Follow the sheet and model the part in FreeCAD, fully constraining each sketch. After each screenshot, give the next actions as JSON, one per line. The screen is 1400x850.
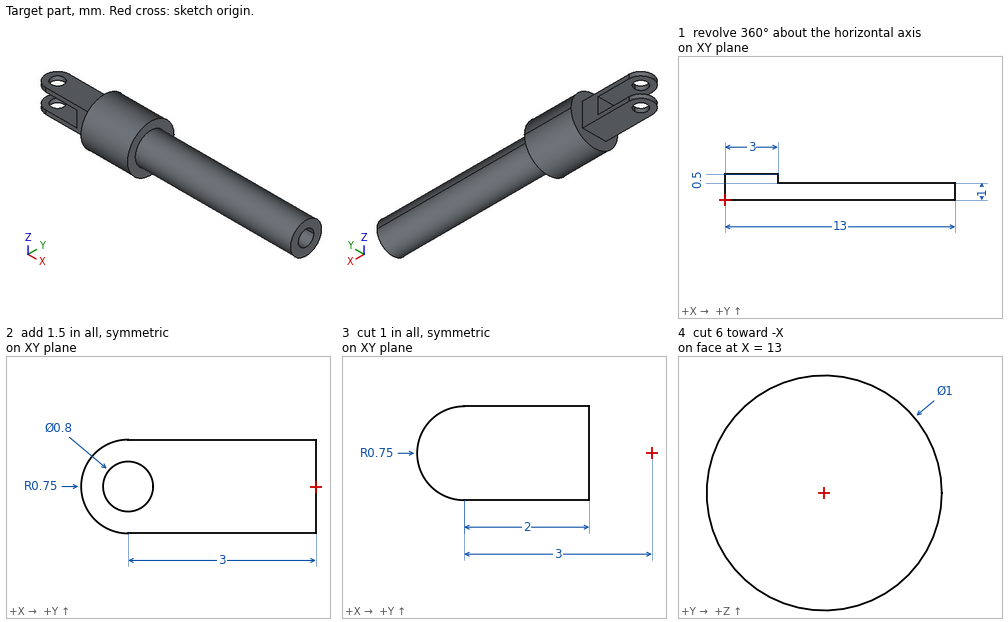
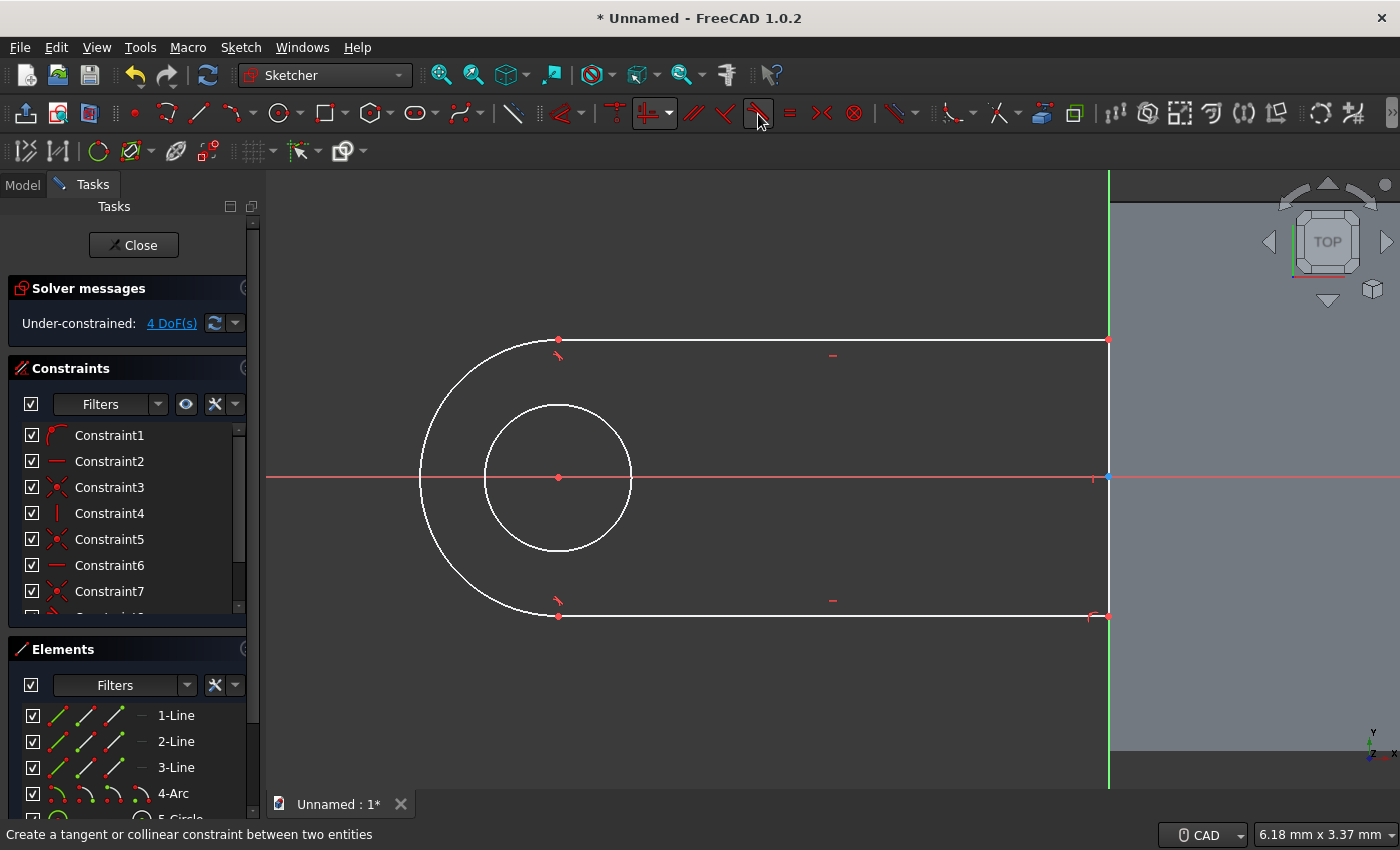
{"action": "left_click", "coordinate": [558, 478]}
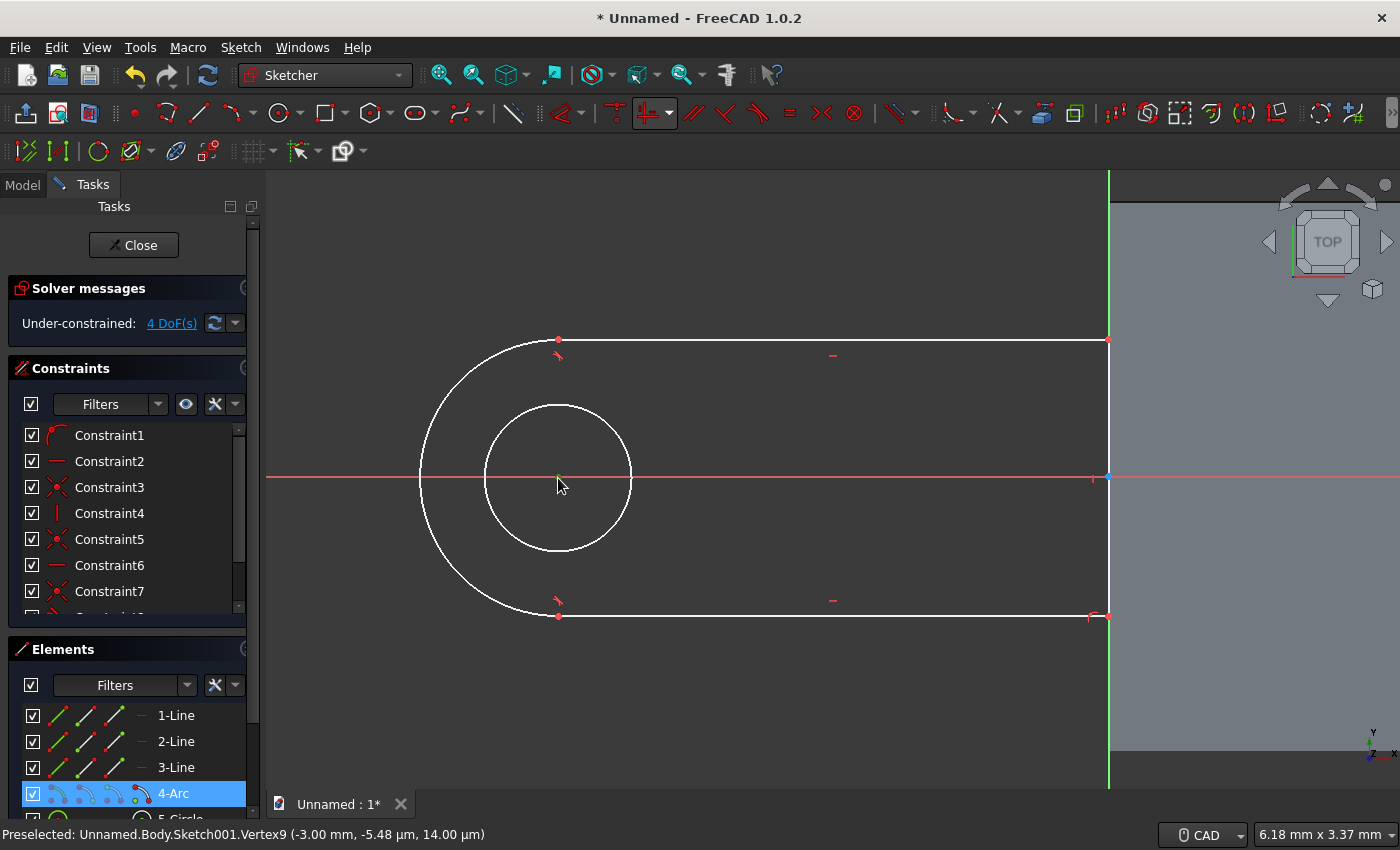
{"action": "left_click", "coordinate": [361, 477]}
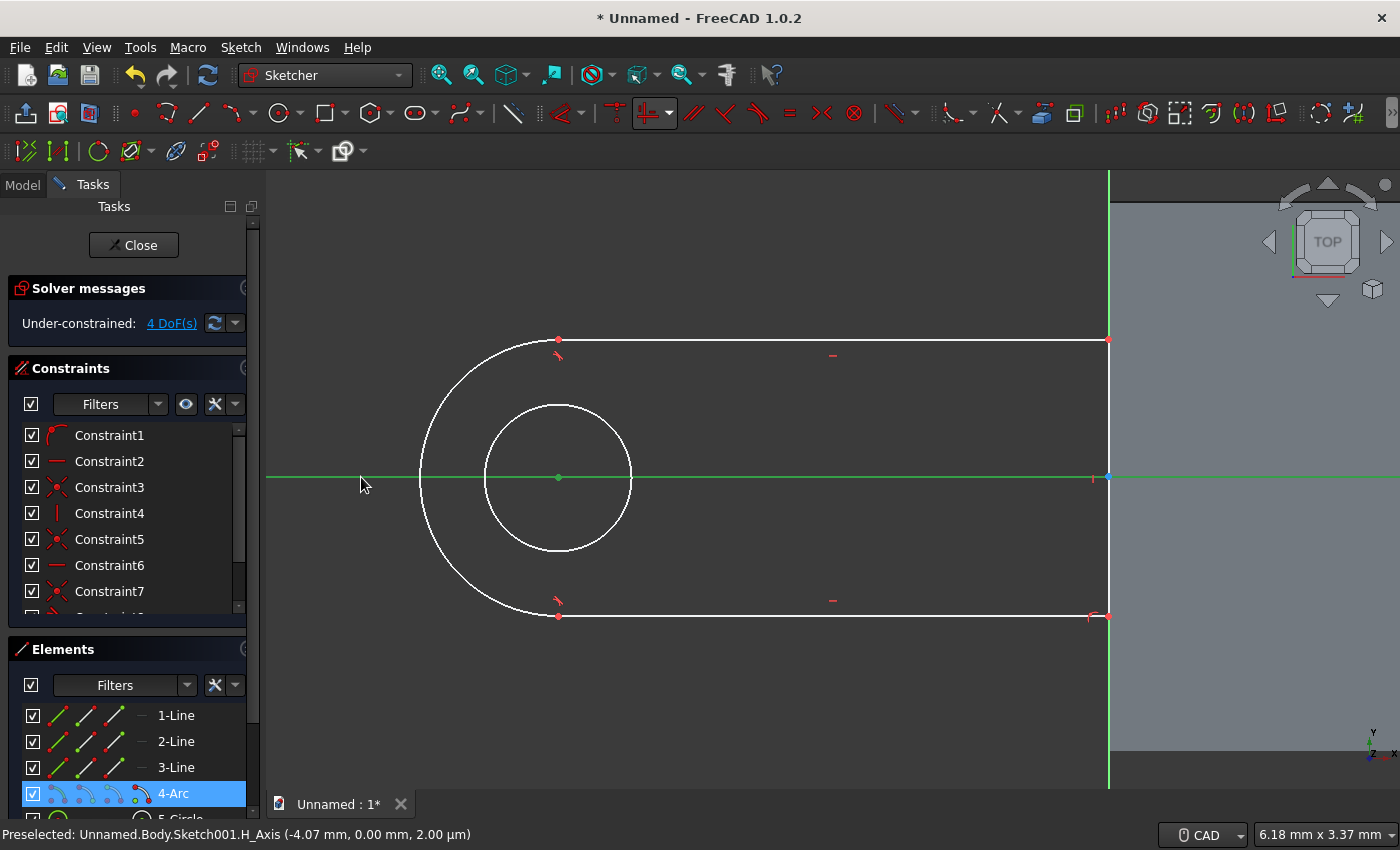
{"action": "left_click", "coordinate": [616, 114]}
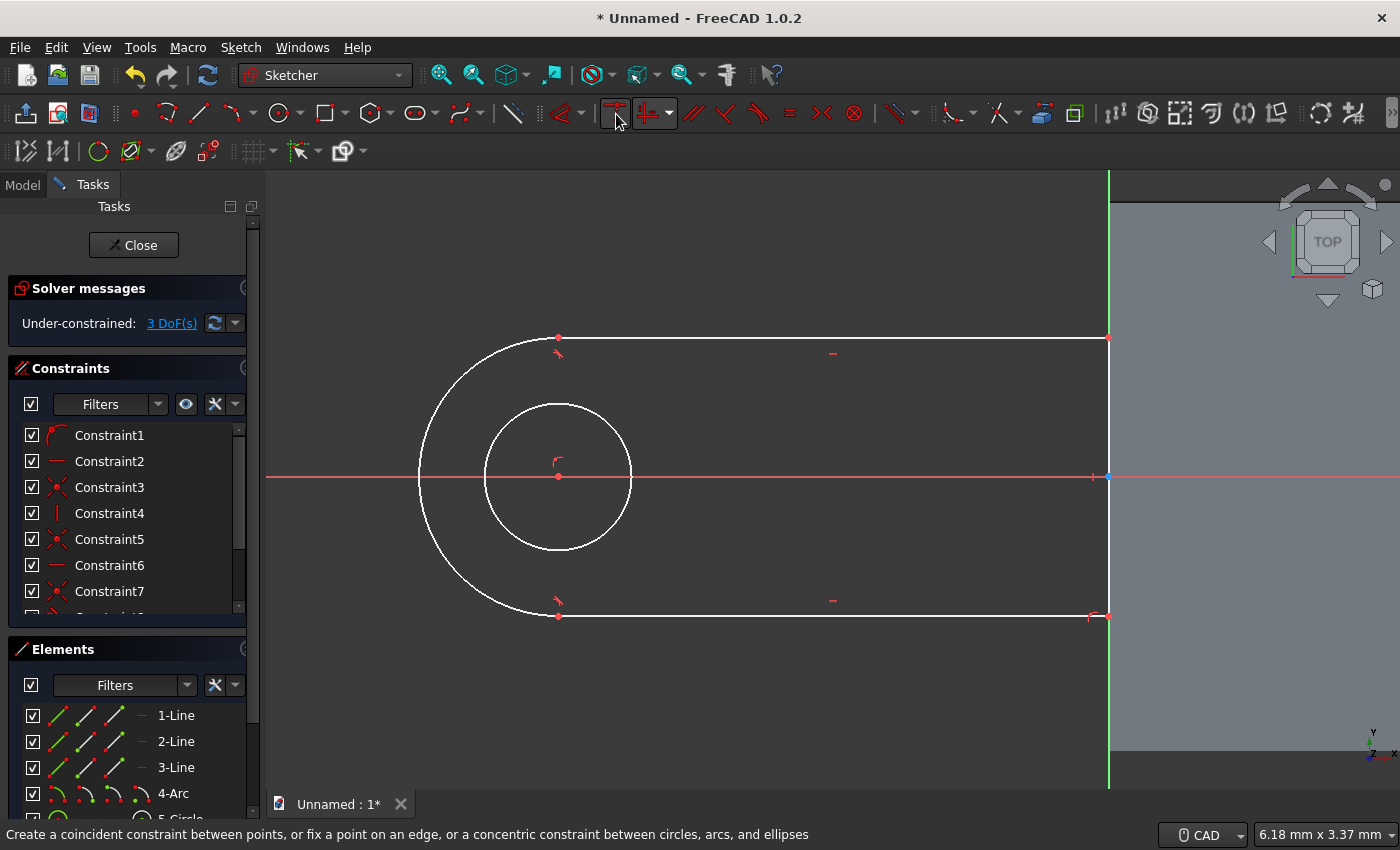
{"action": "left_click", "coordinate": [560, 114]}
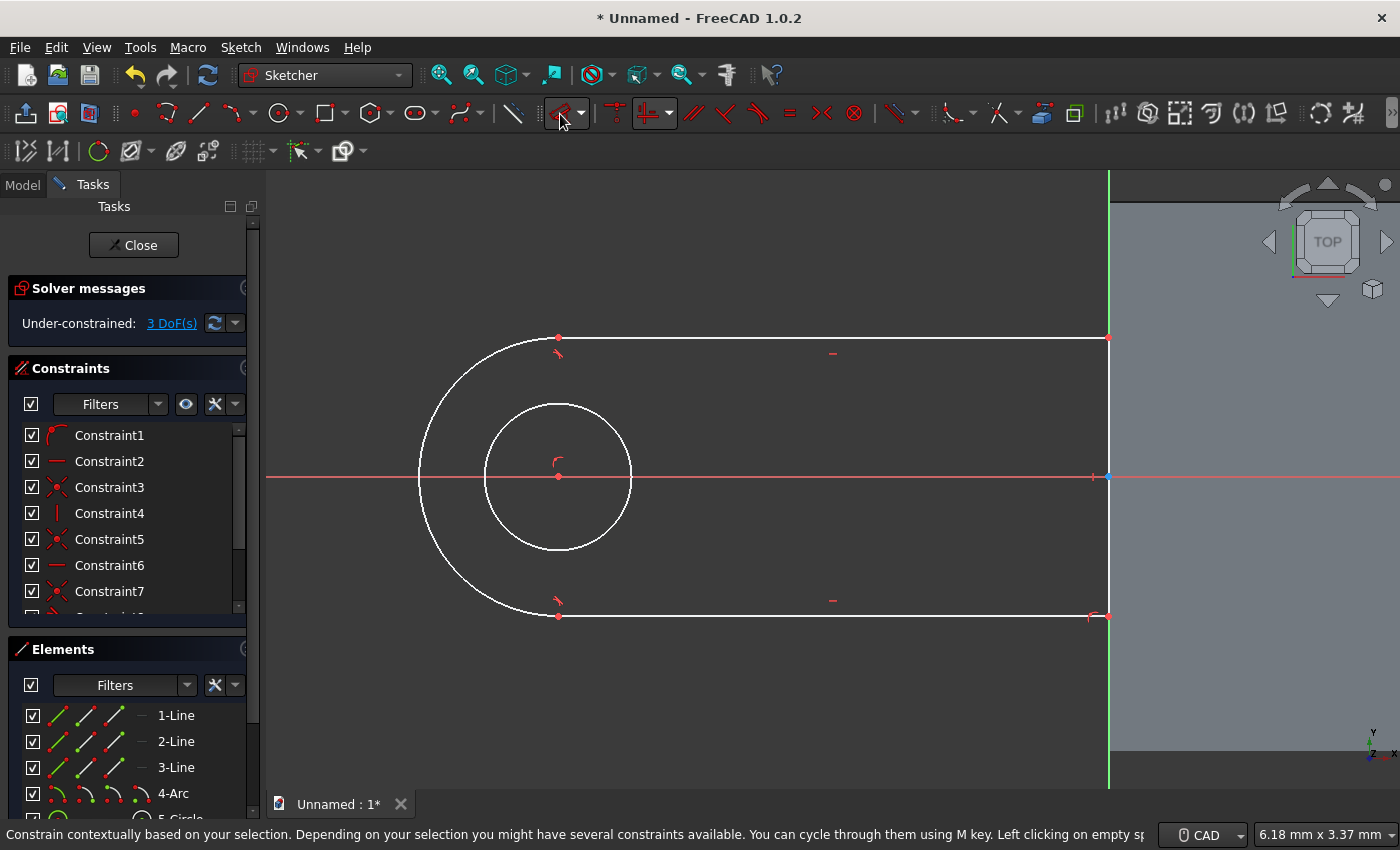
{"action": "left_click", "coordinate": [446, 395]}
{"action": "left_click", "coordinate": [420, 376]}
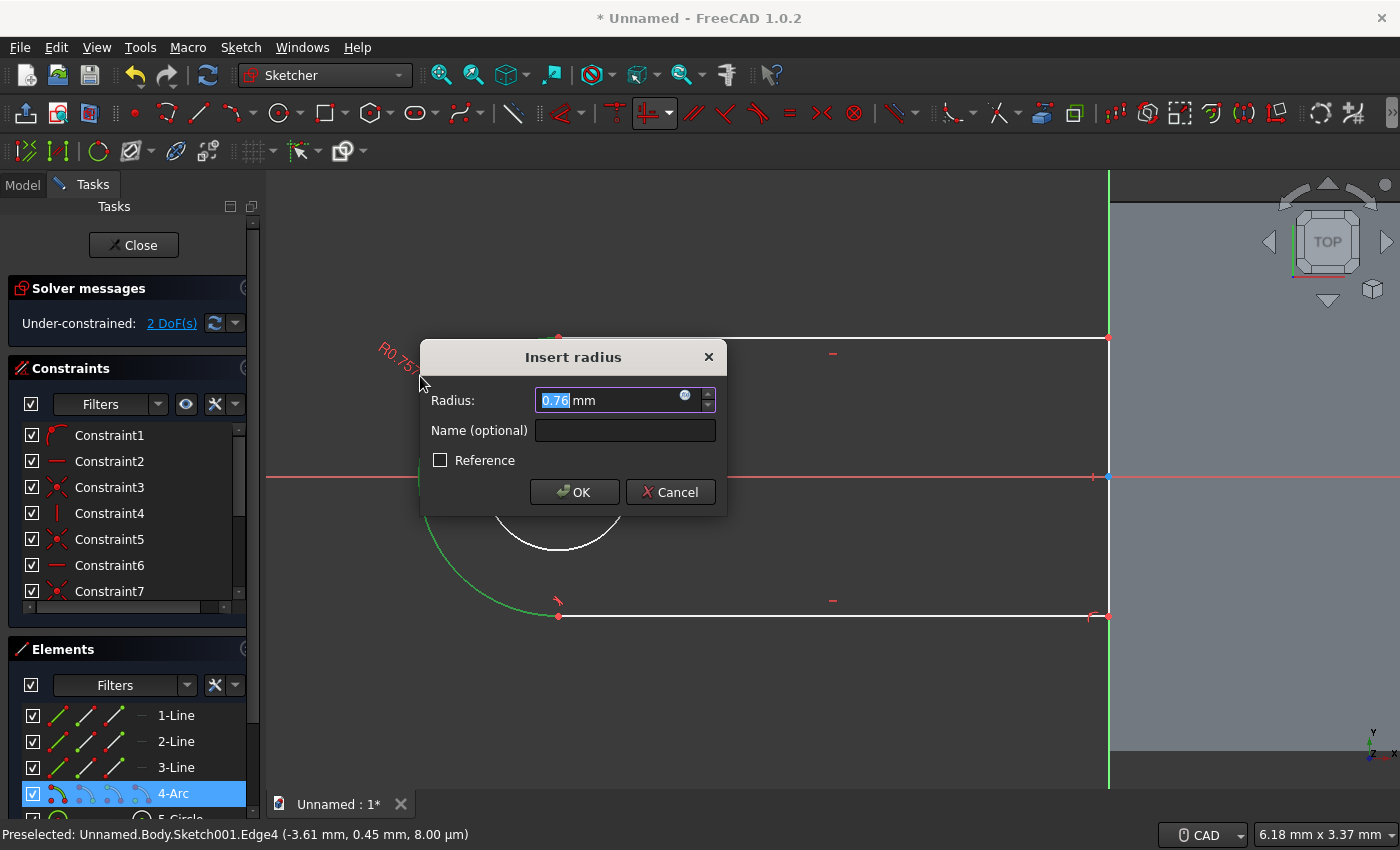
{"action": "type", "text": "0.75"}
{"action": "key", "text": "Return"}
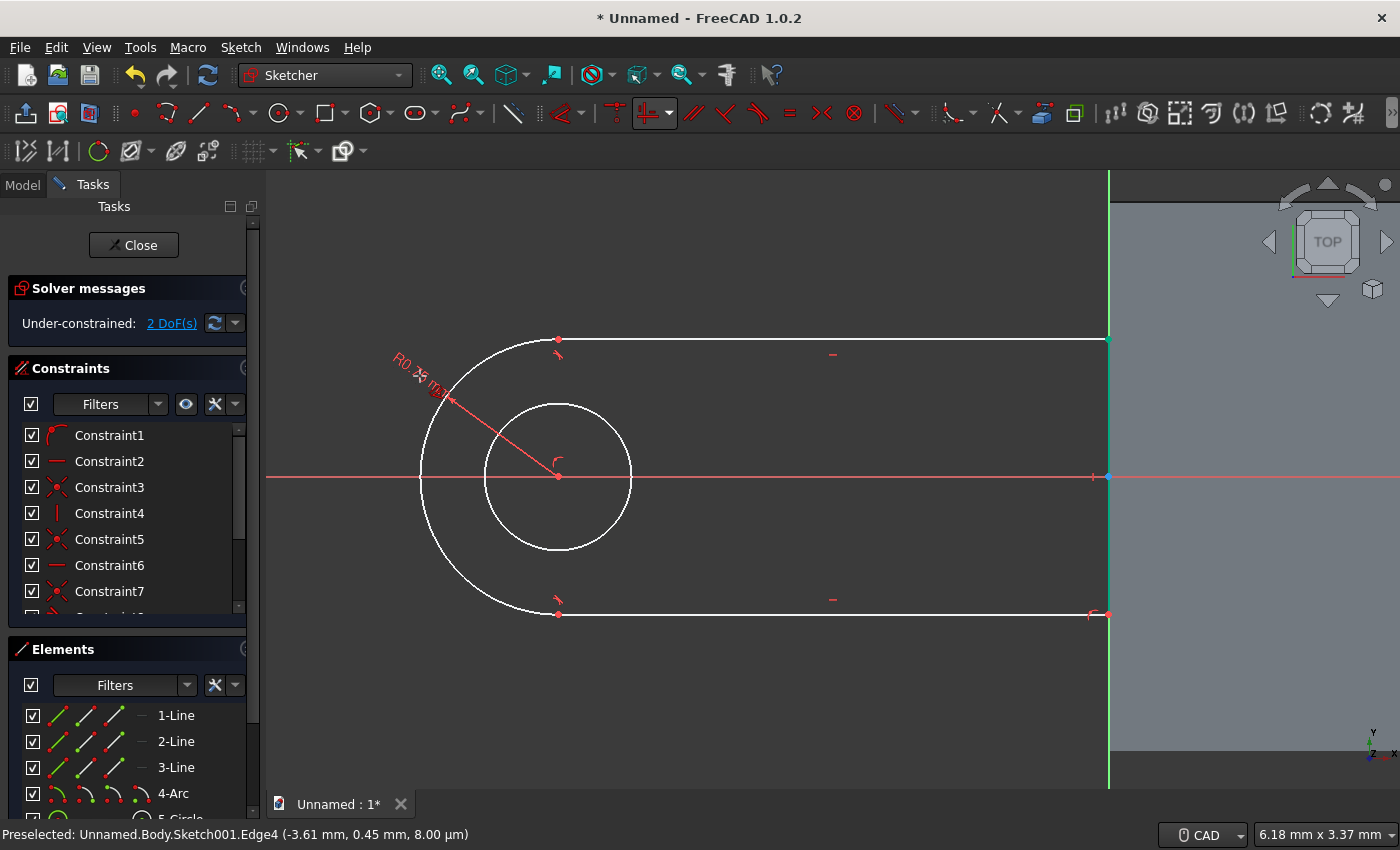
{"action": "left_click", "coordinate": [610, 425]}
{"action": "left_click", "coordinate": [633, 402]}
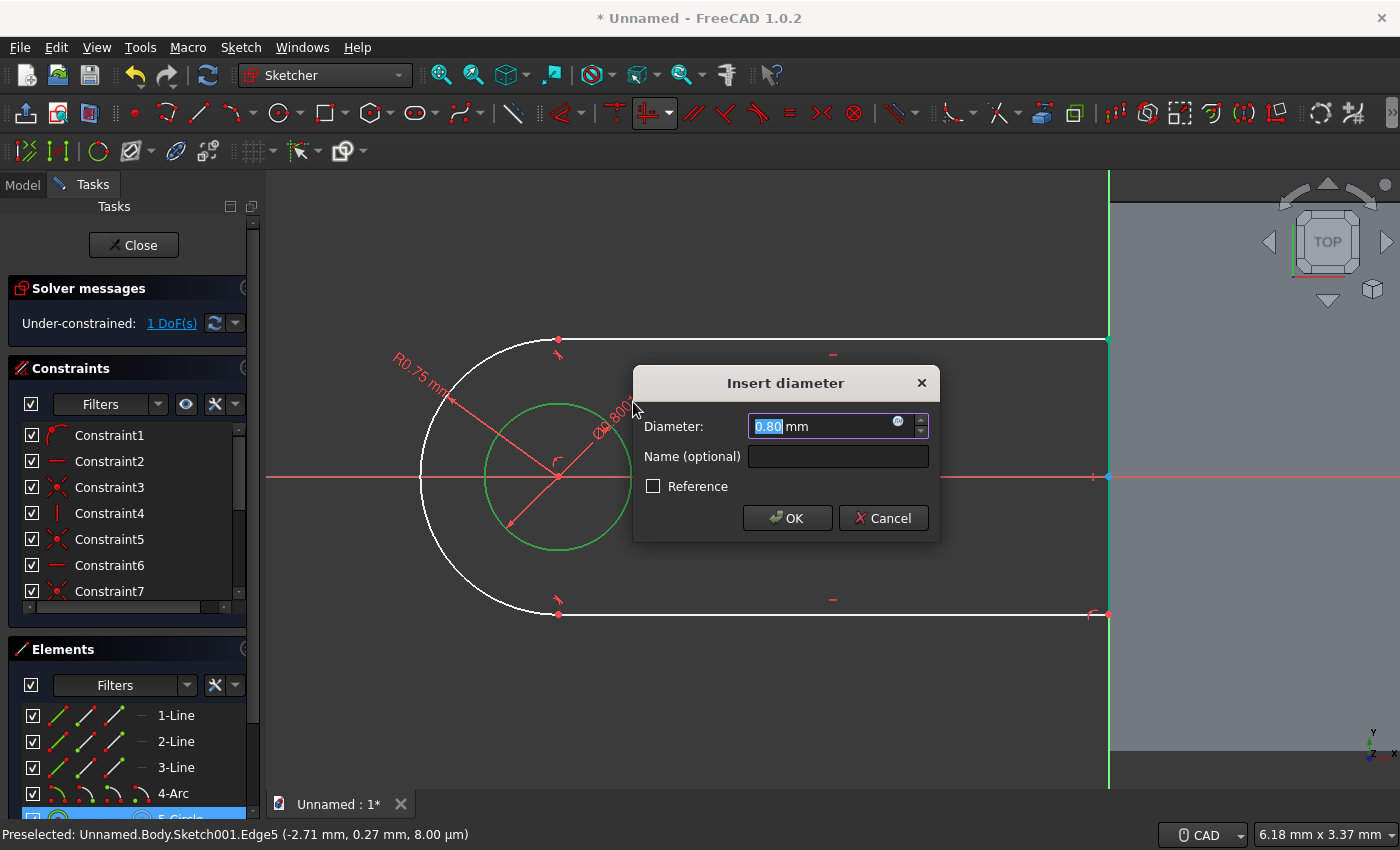
{"action": "type", "text": "0.8"}
{"action": "key", "text": "Return"}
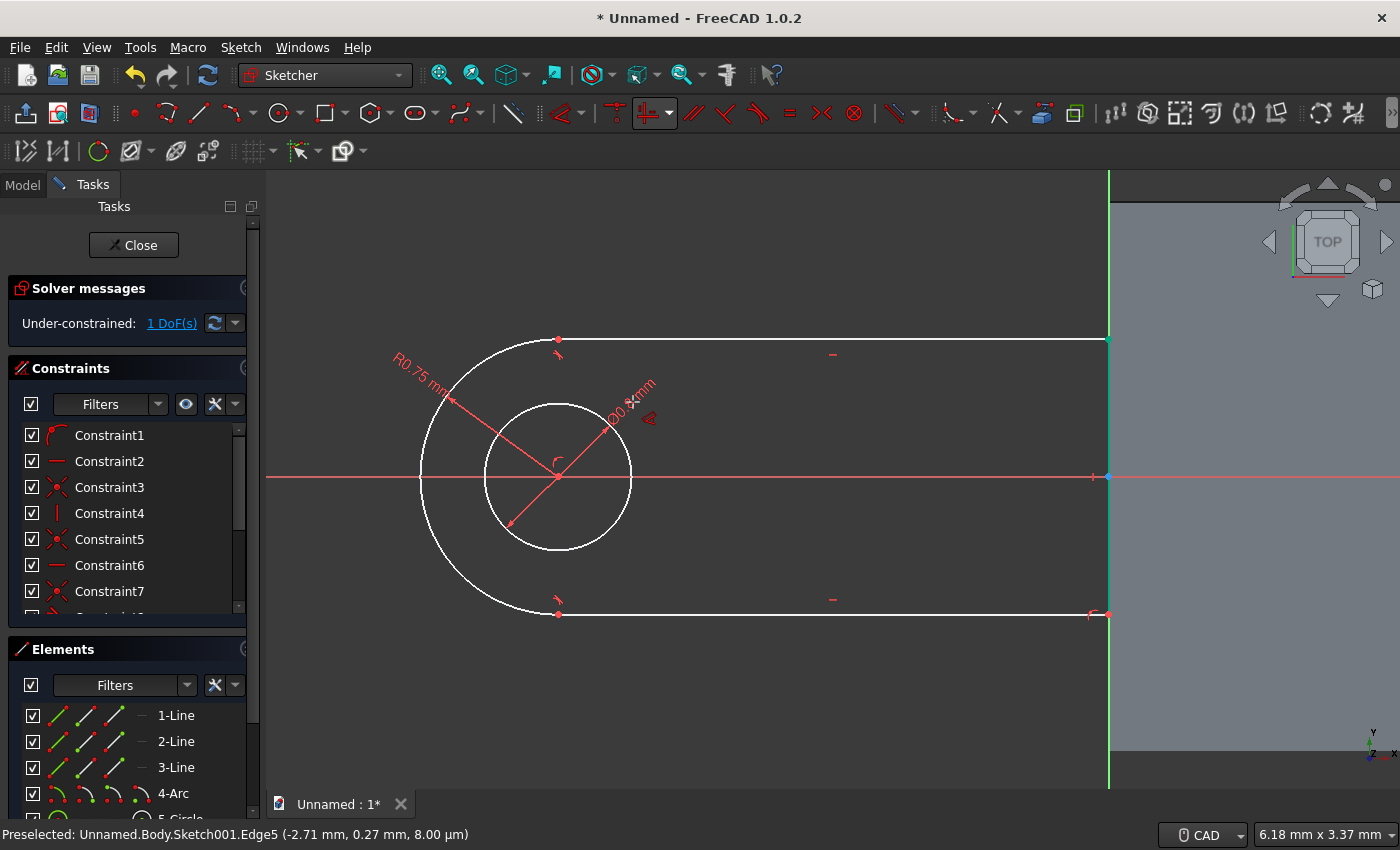
{"action": "left_click", "coordinate": [723, 615]}
{"action": "left_click", "coordinate": [834, 649]}